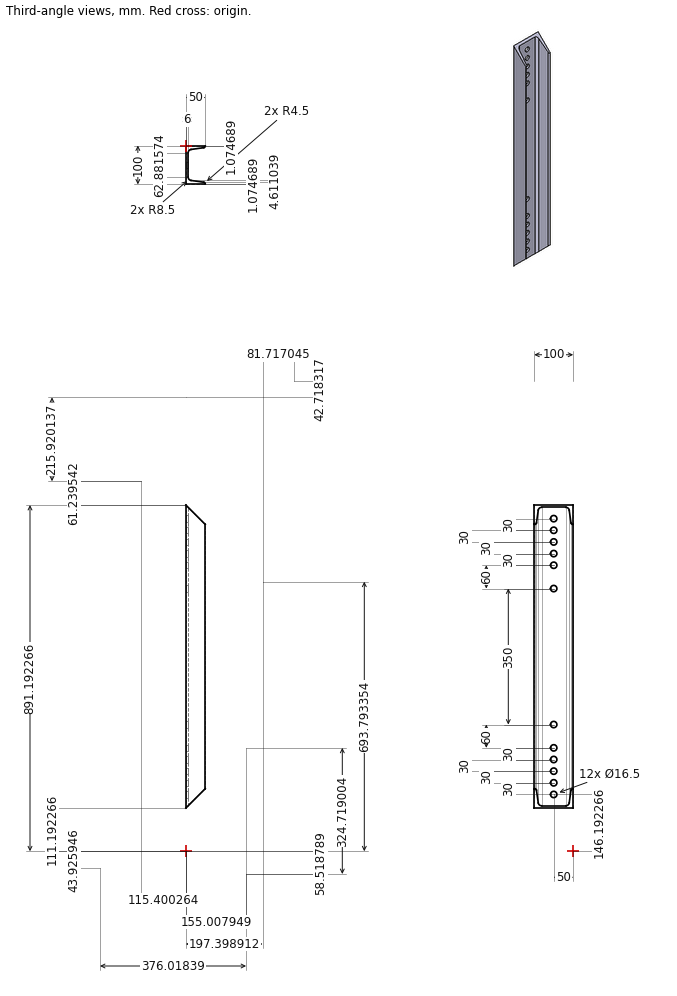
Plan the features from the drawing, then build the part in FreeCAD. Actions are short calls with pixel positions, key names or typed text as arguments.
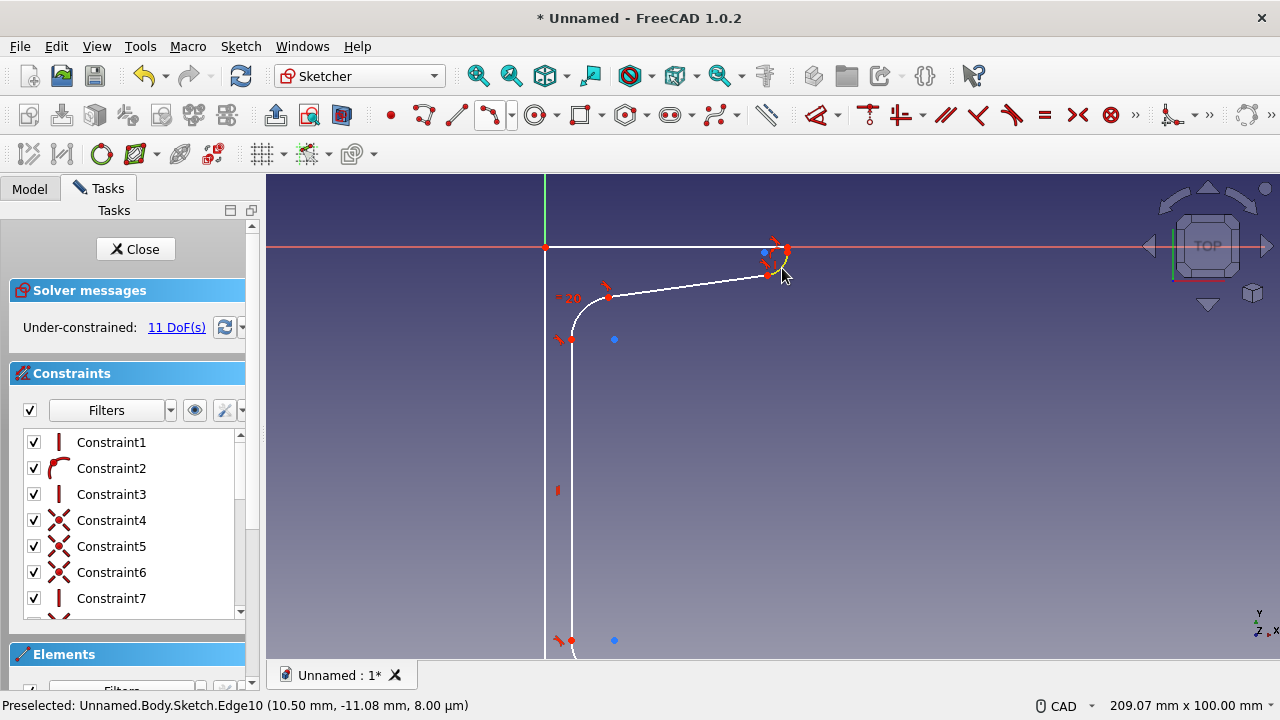
click(782, 268)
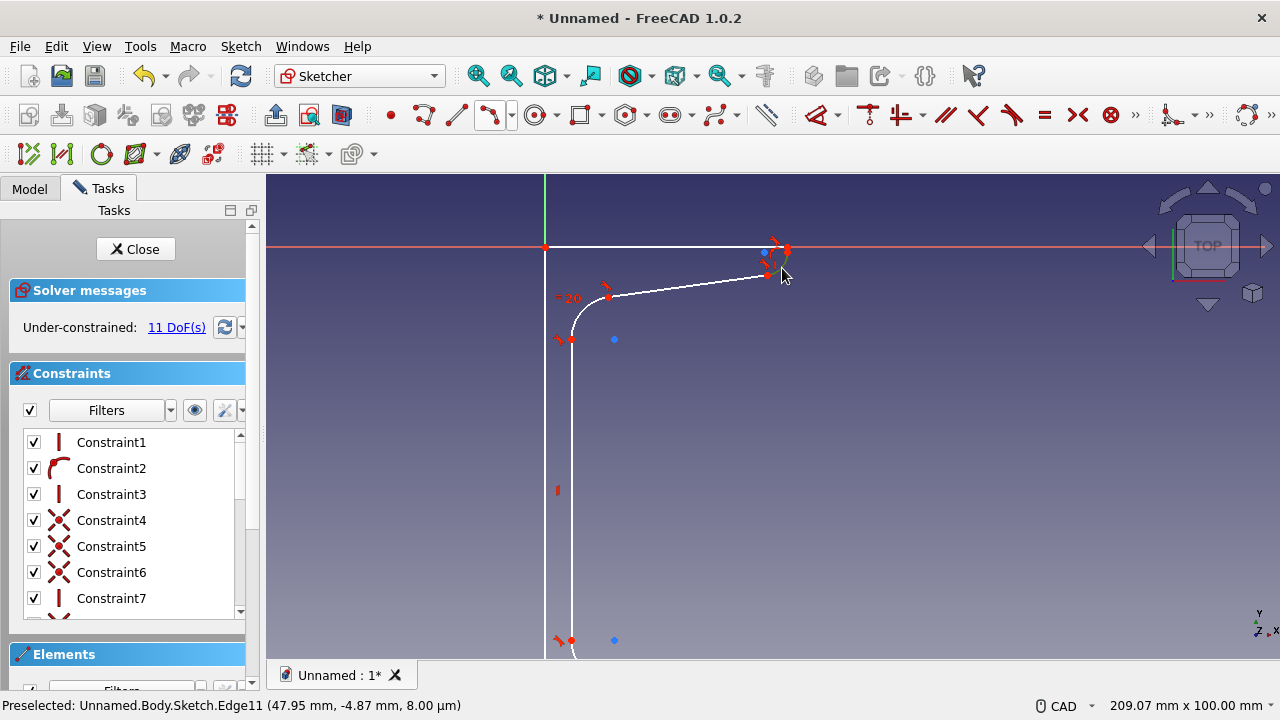
scroll(782, 267, down, 2)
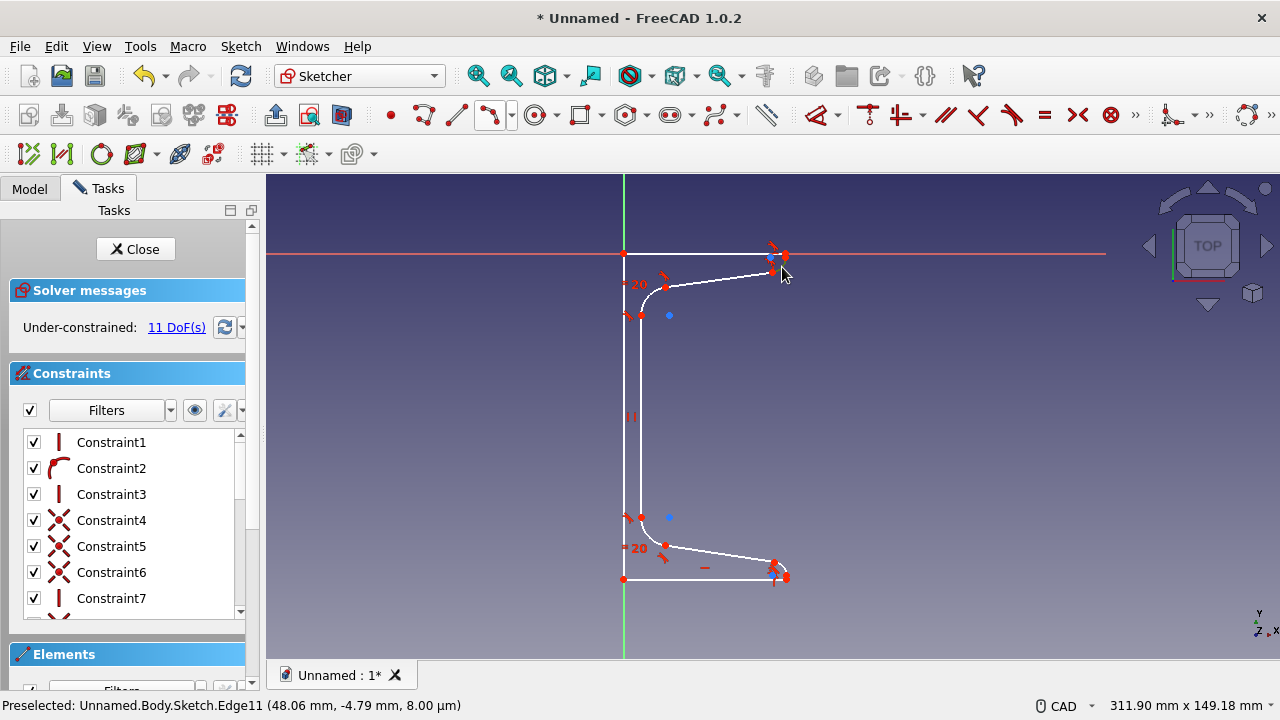
scroll(783, 567, up, 2)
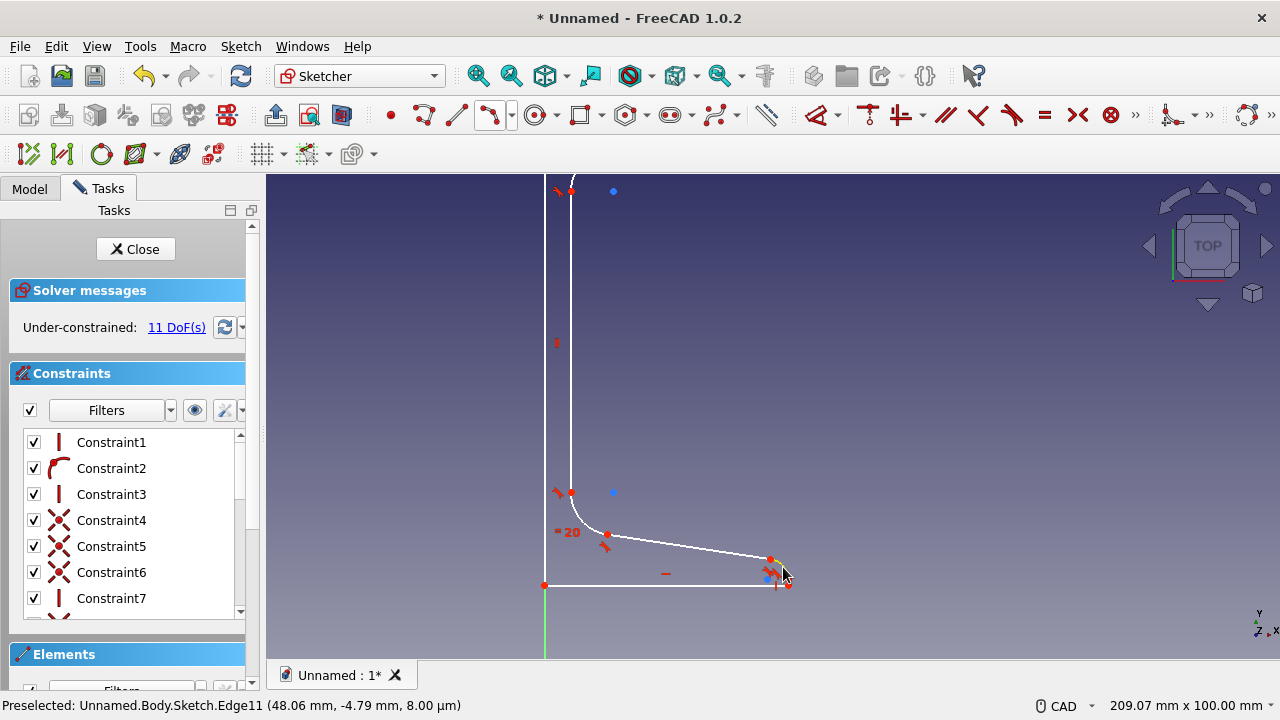
click(783, 566)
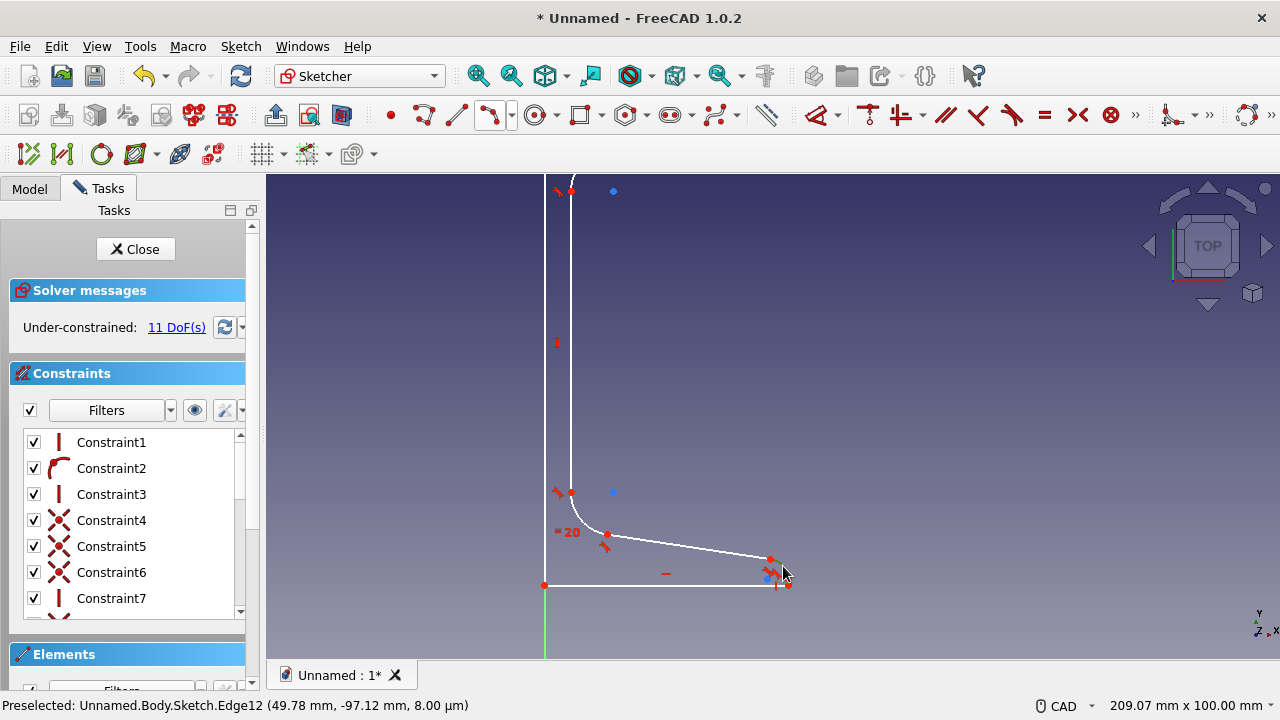
click(1045, 116)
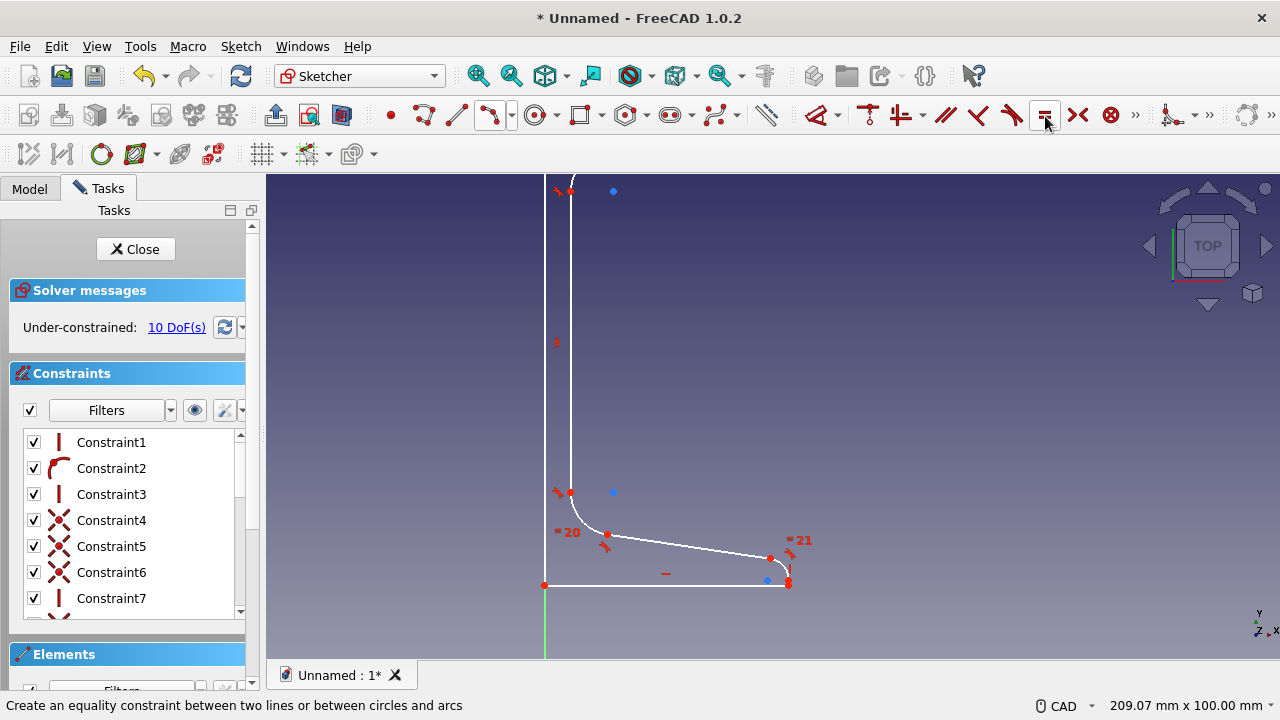
click(575, 510)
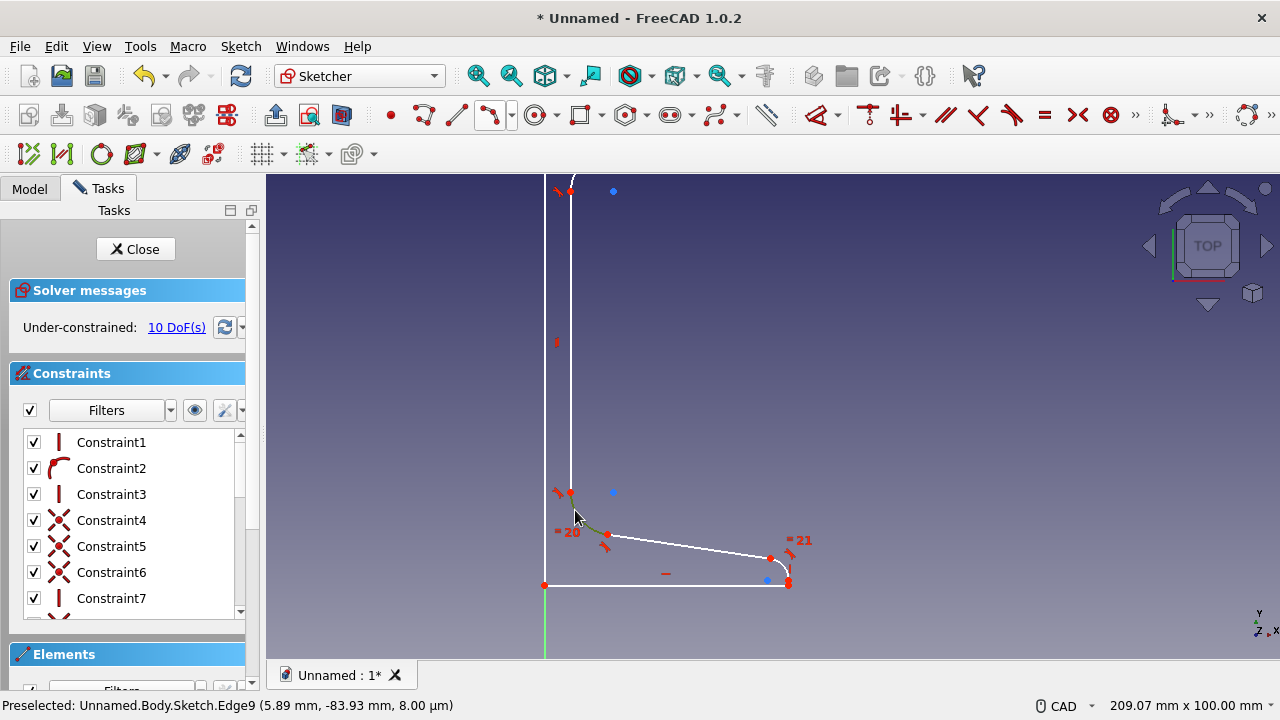
key(k)
key(r)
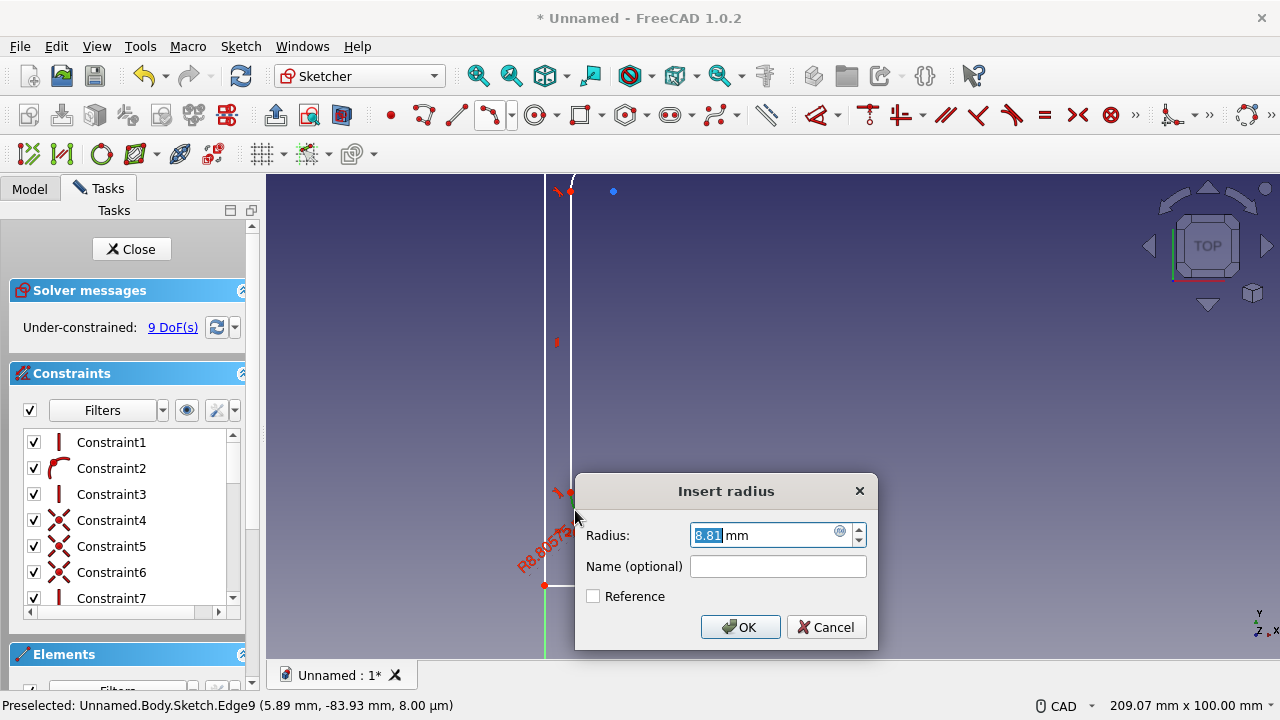
text(8.5)
key(Return)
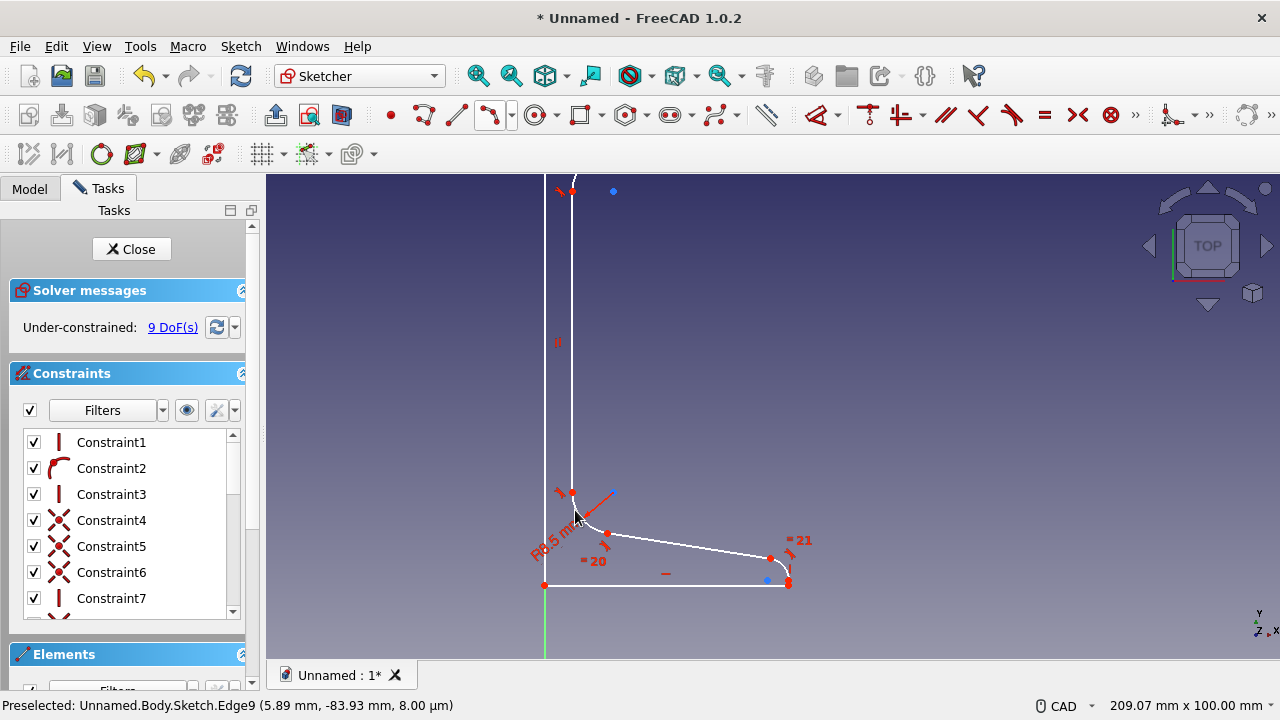
scroll(783, 568, down, 2)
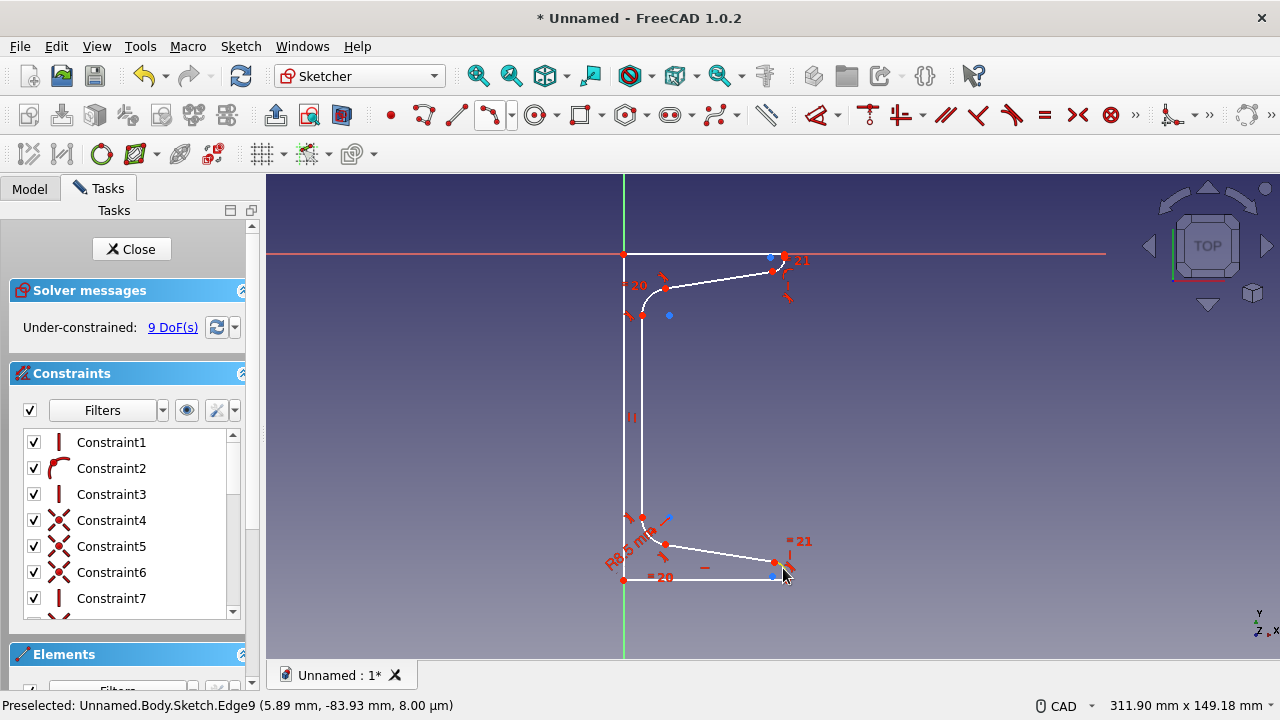
scroll(778, 270, up, 5)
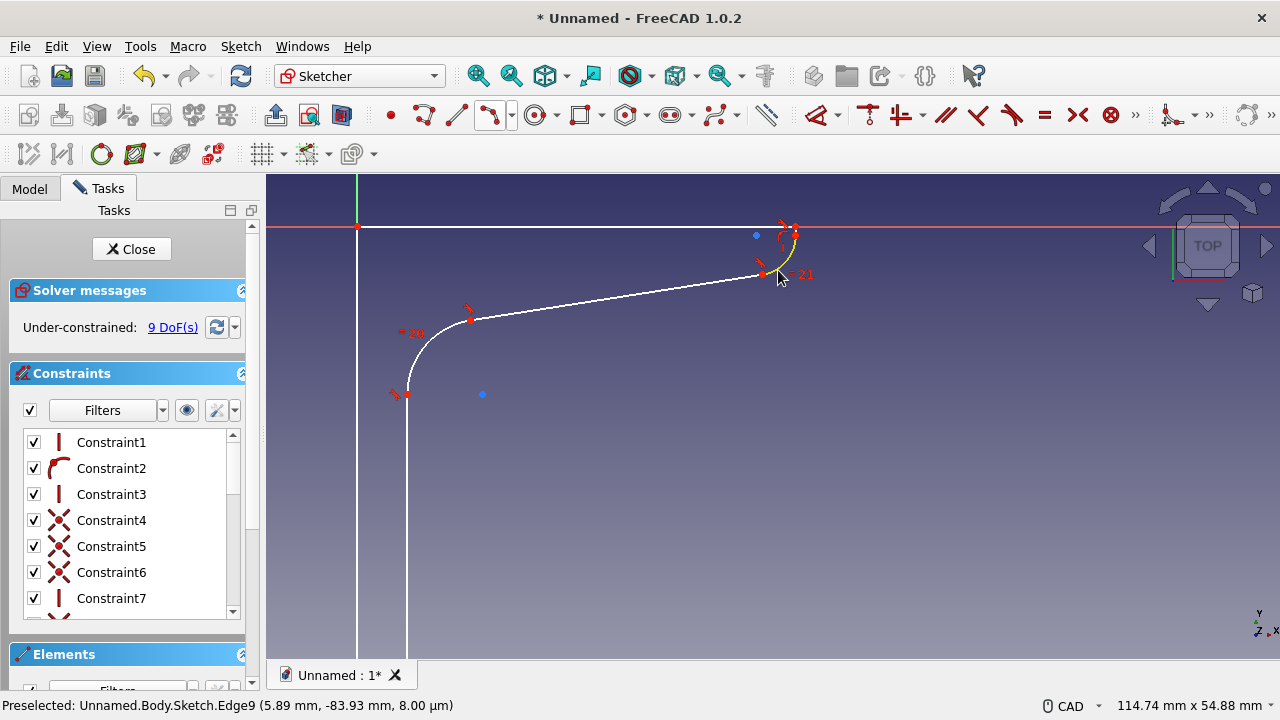
click(778, 269)